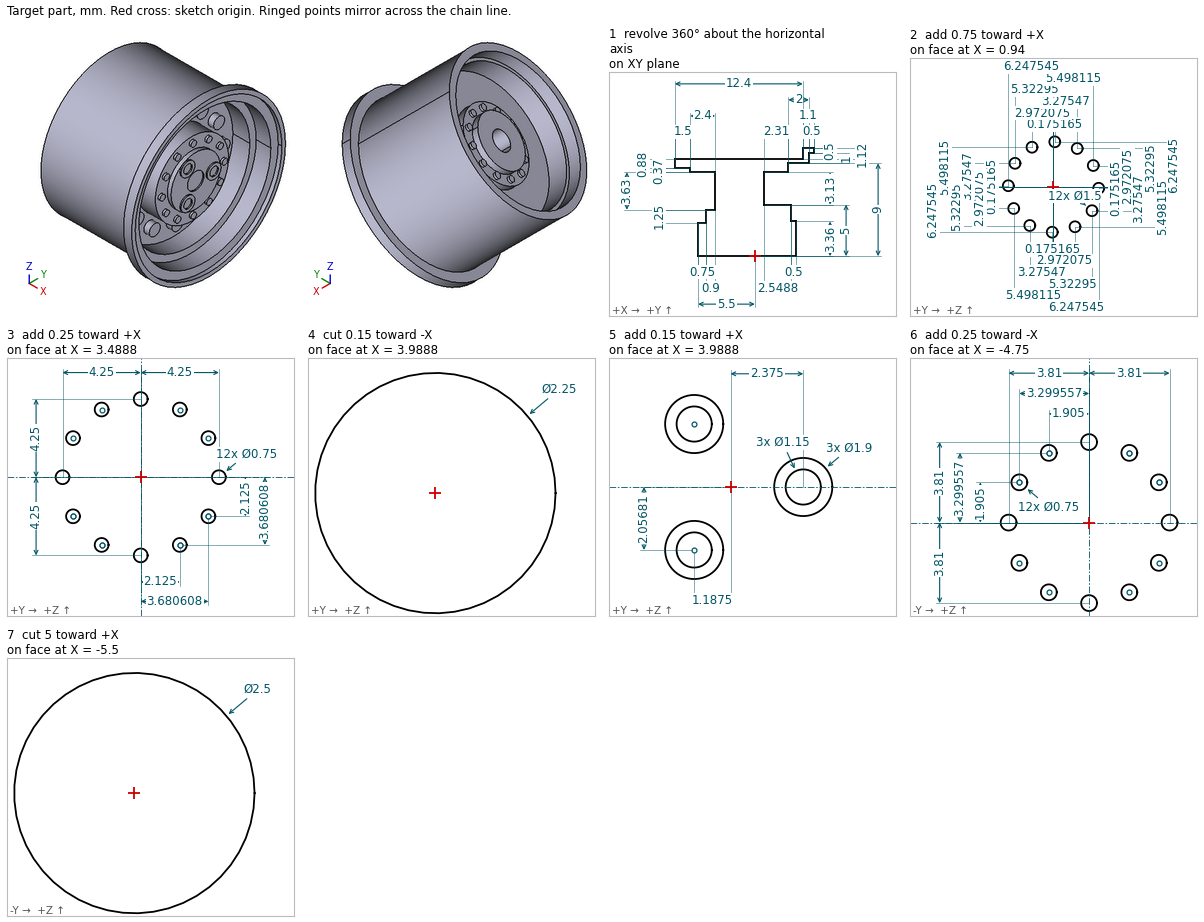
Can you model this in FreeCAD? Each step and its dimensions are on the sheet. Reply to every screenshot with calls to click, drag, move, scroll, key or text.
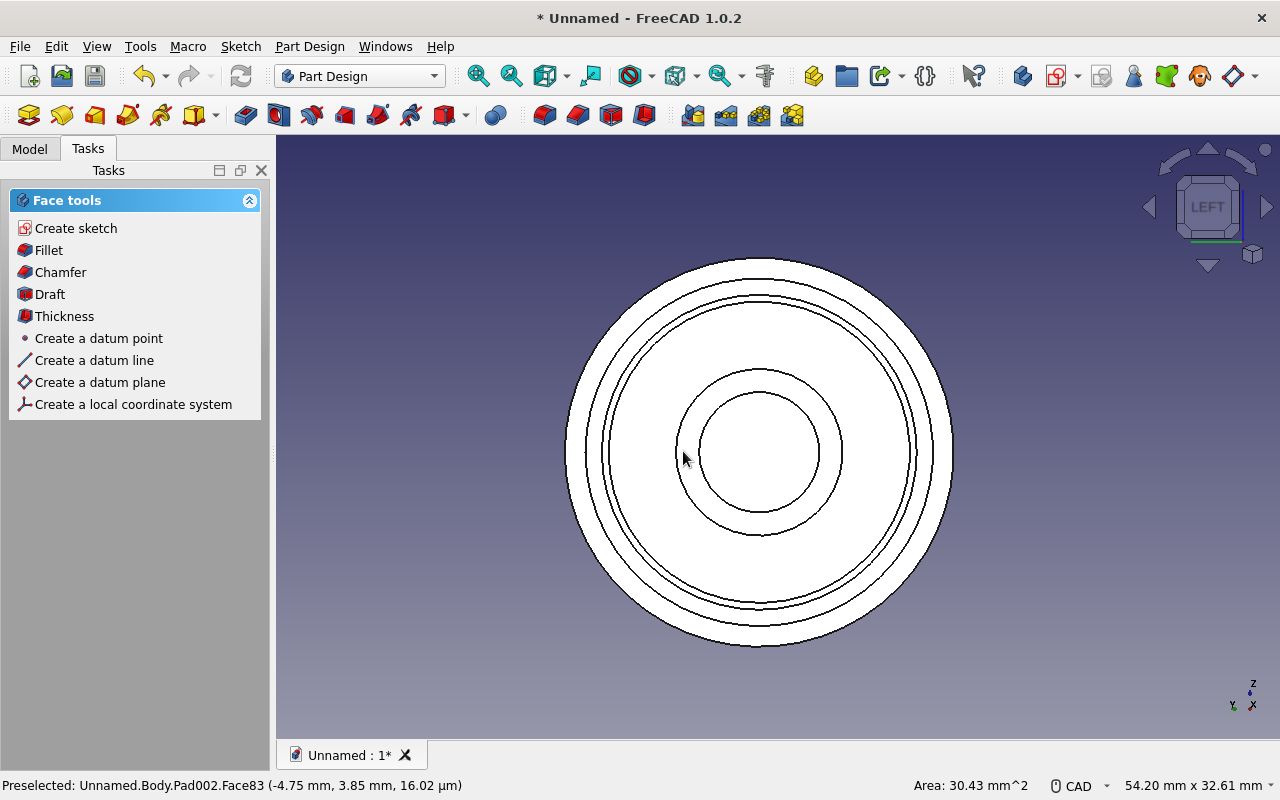
click(1056, 76)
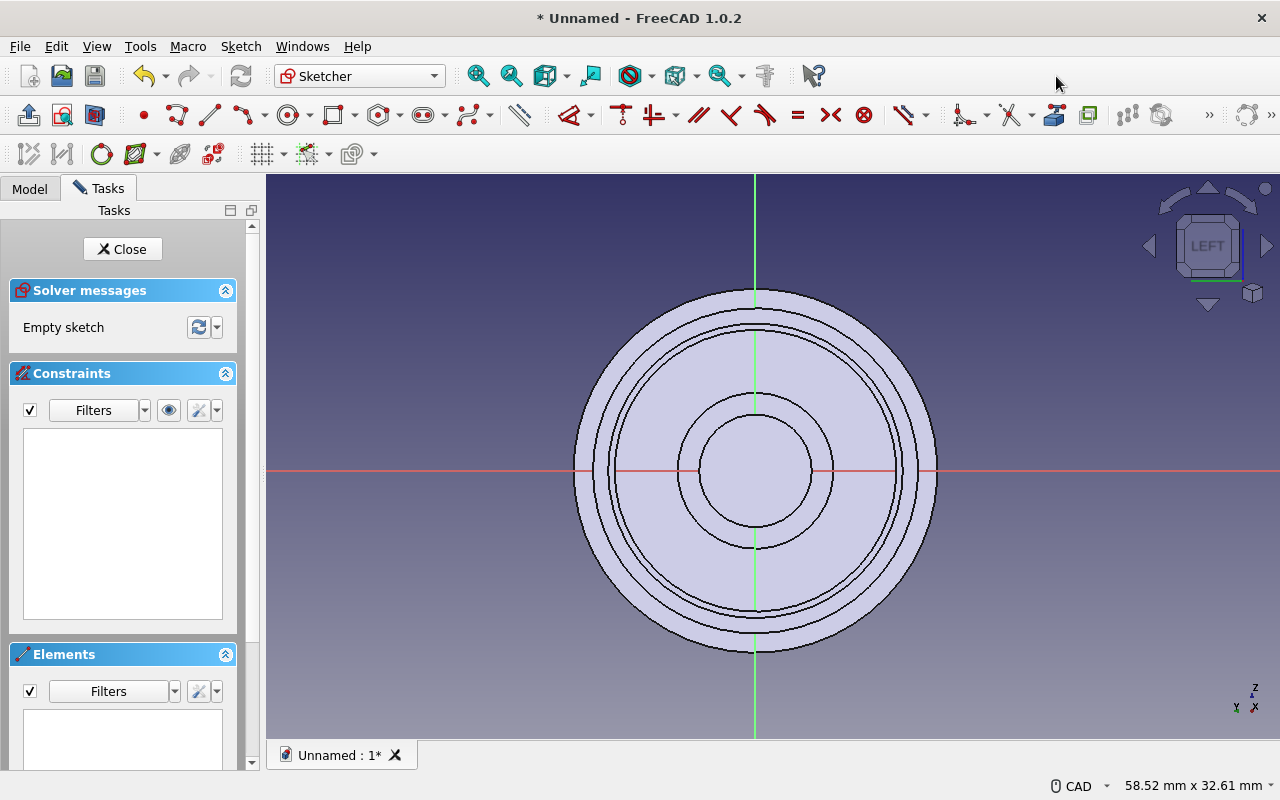
scroll(785, 479, up, 5)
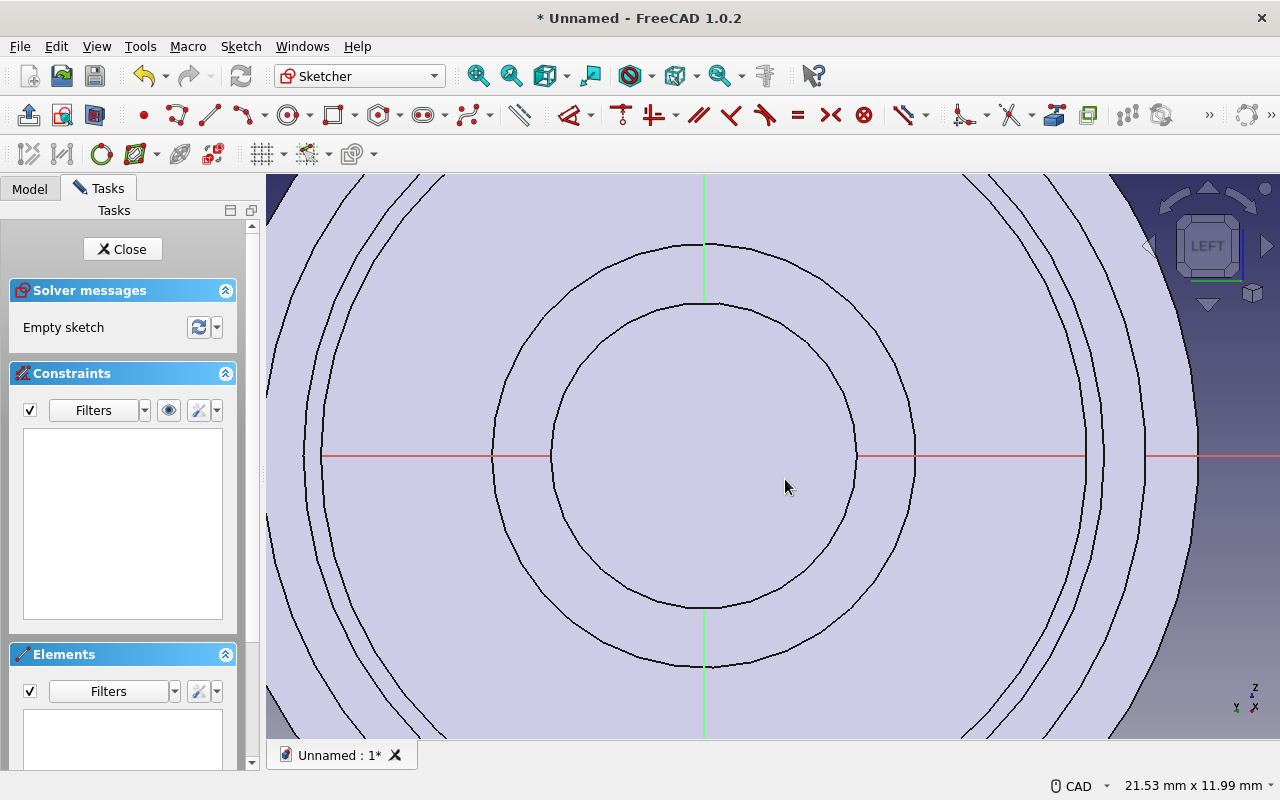
click(288, 116)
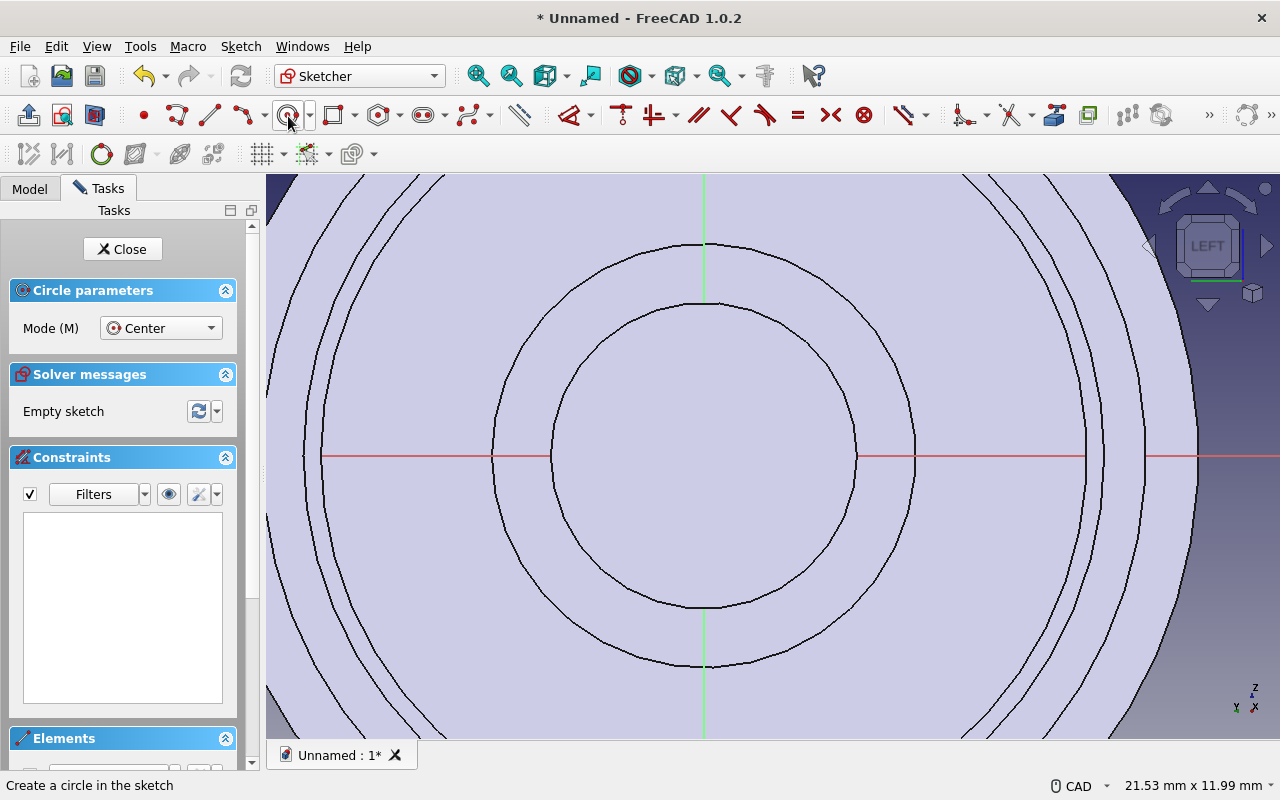
scroll(524, 456, up, 2)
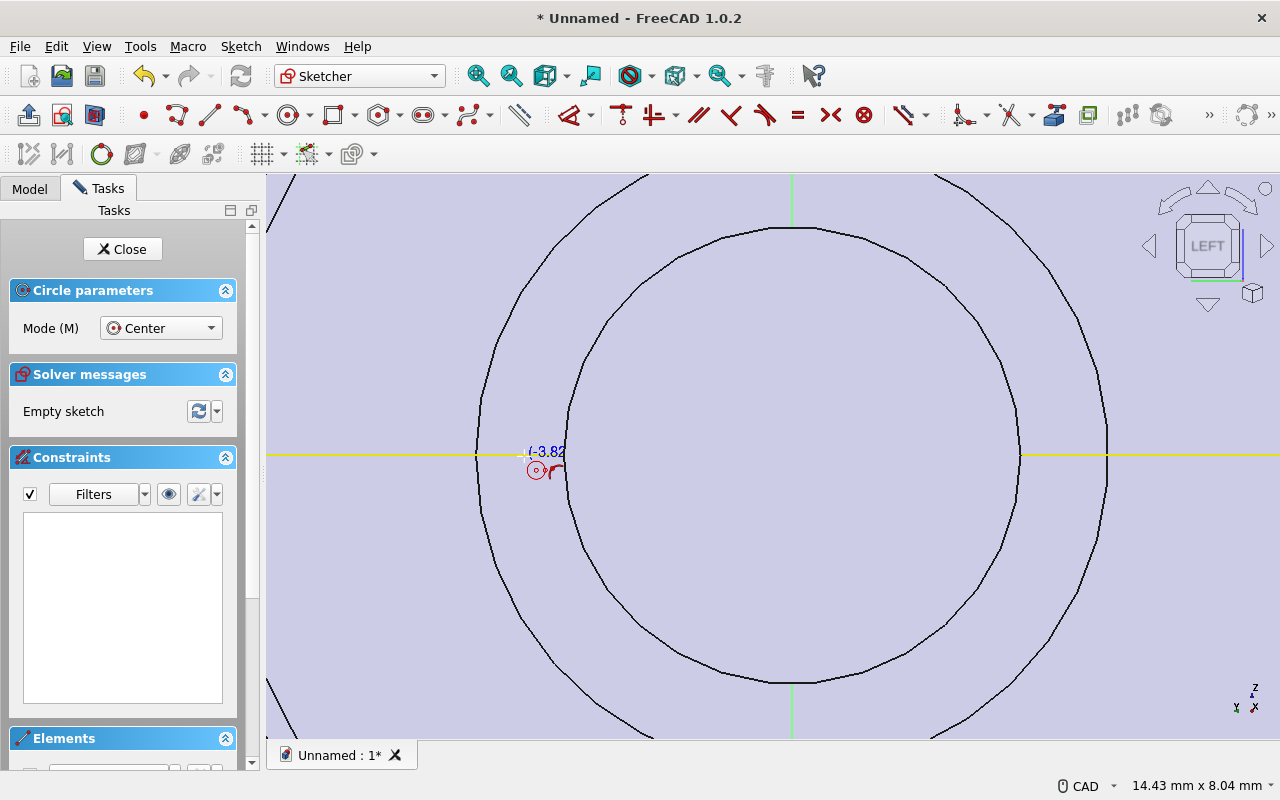
click(524, 455)
move(543, 437)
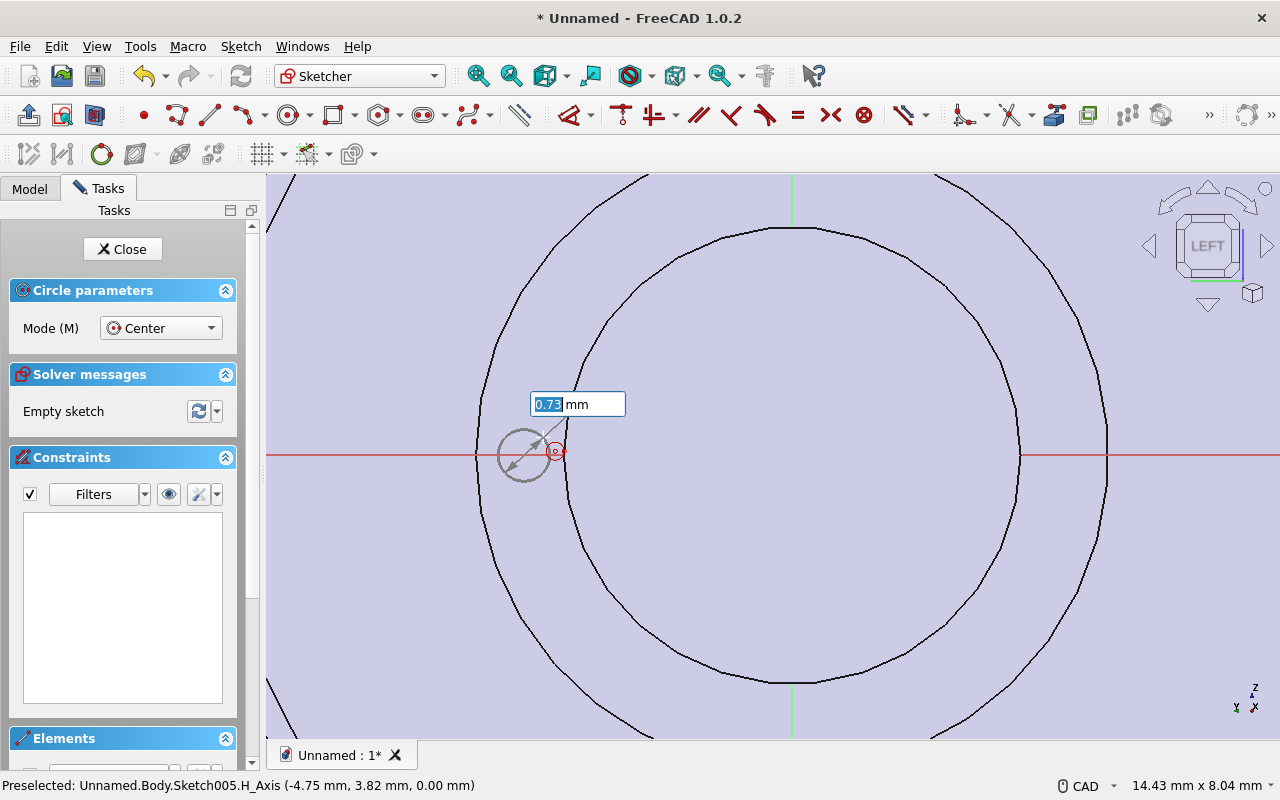
text(0.75)
key(Return)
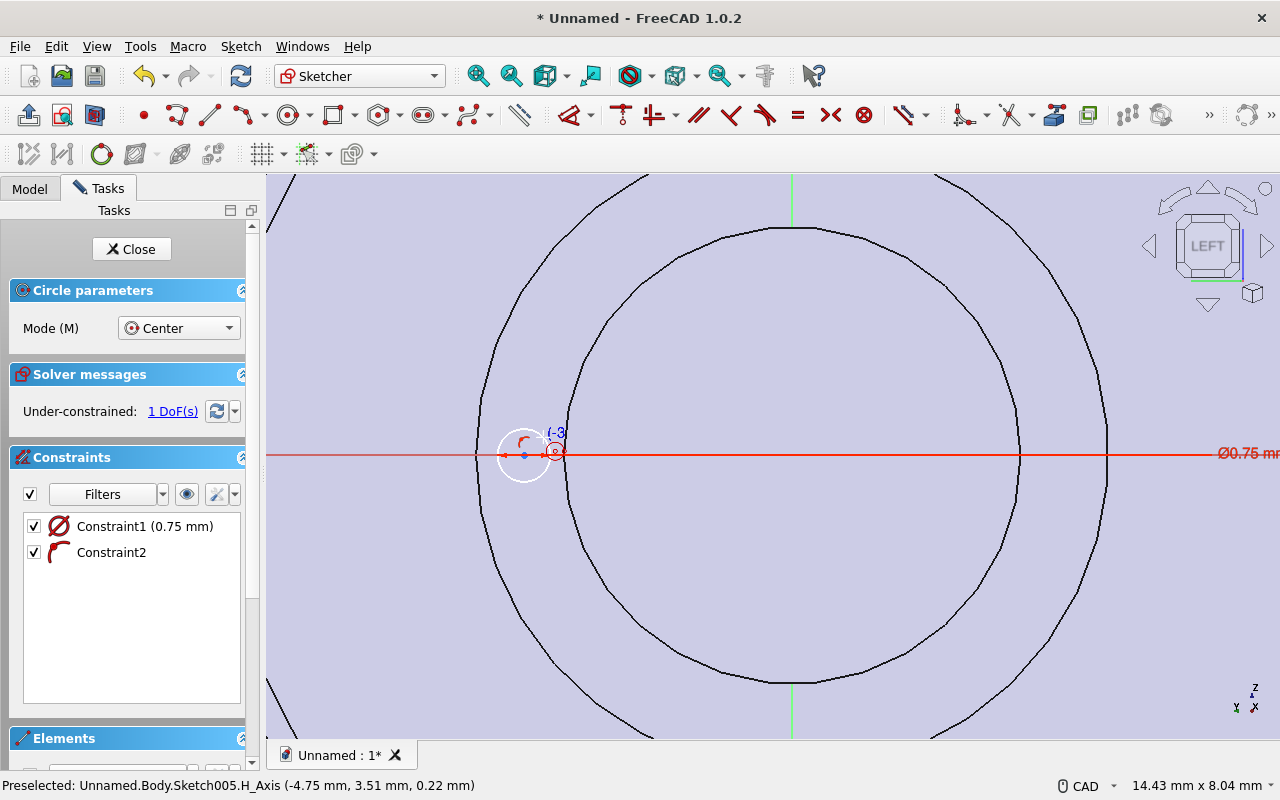
click(560, 322)
move(579, 303)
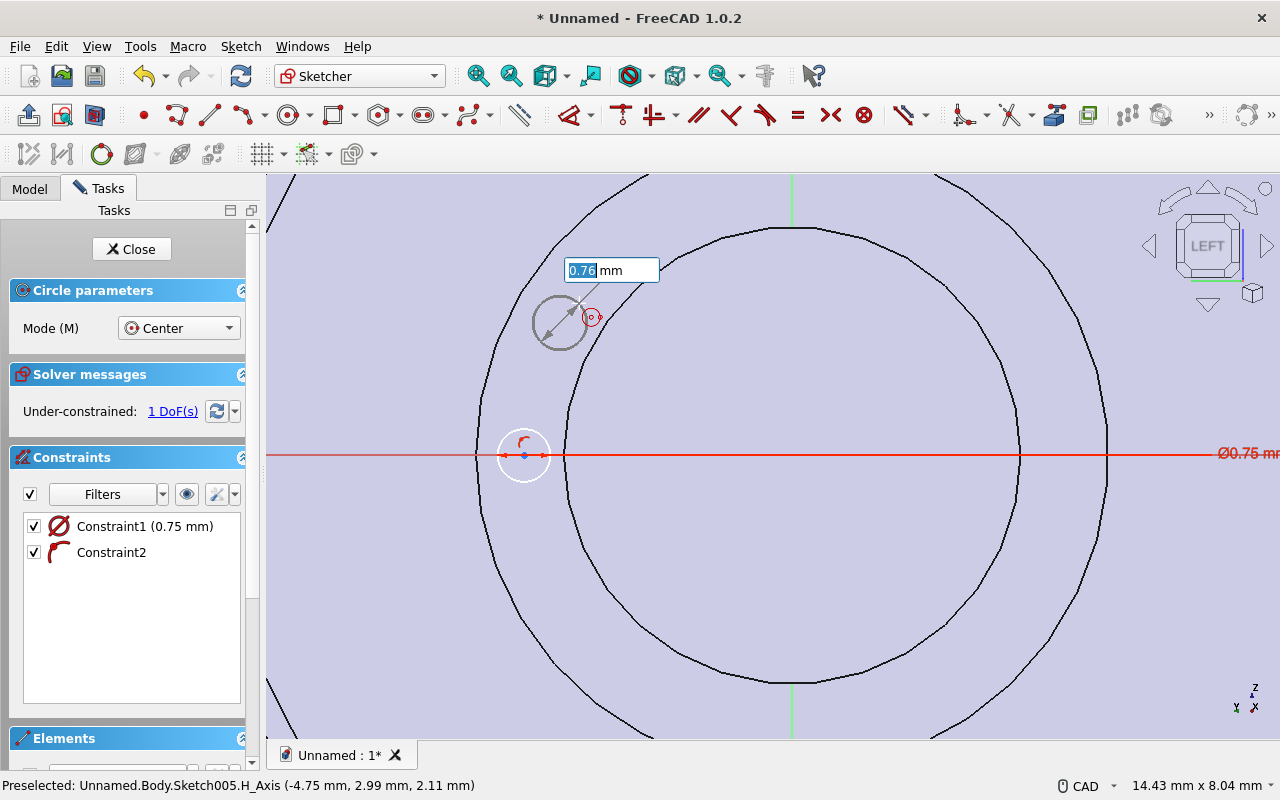
text(0.75)
key(Return)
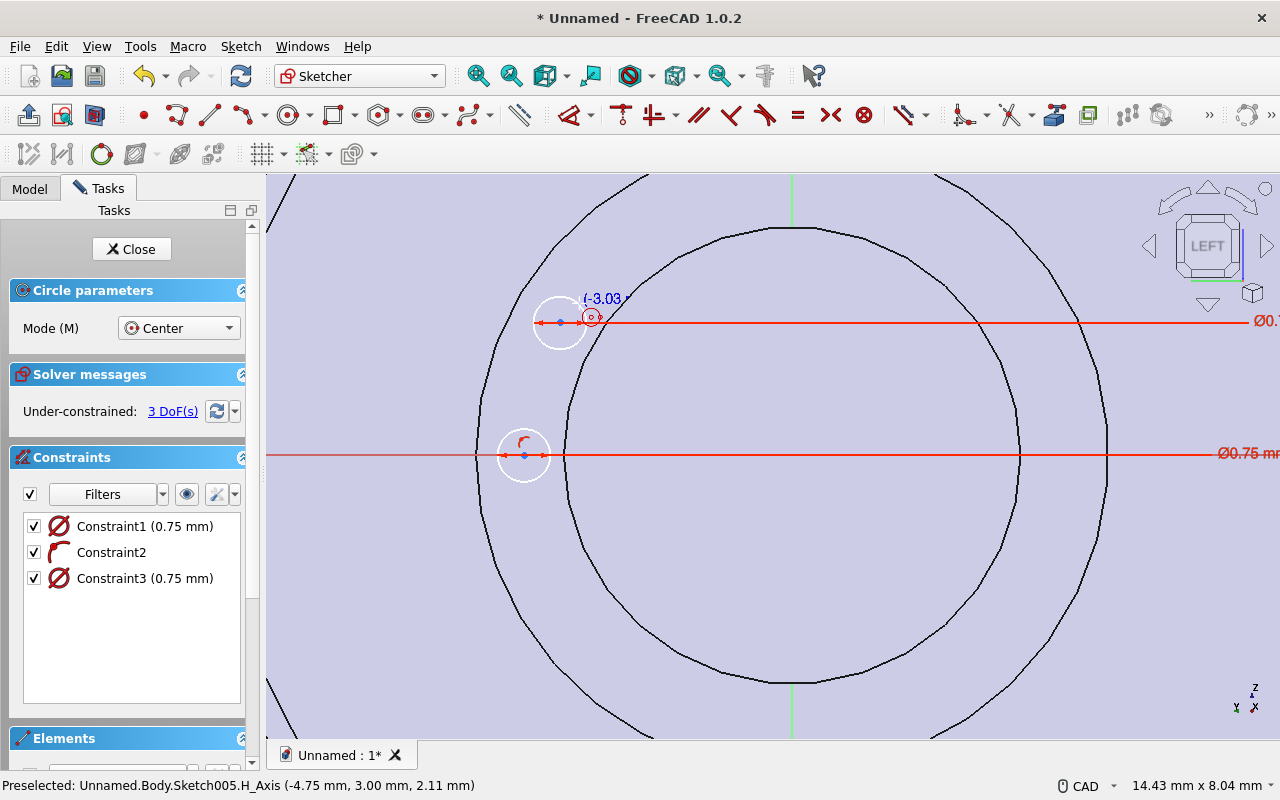
click(658, 224)
move(677, 205)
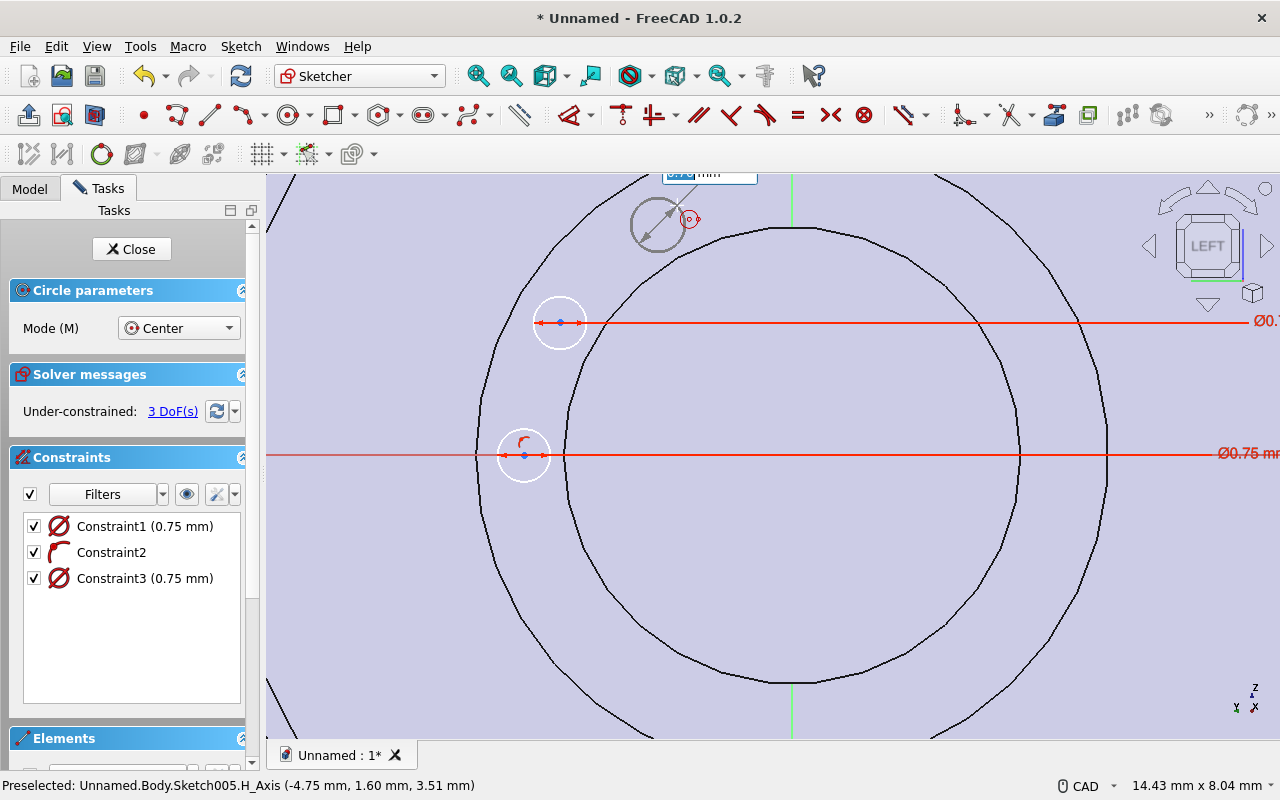
text(0.75)
key(Return)